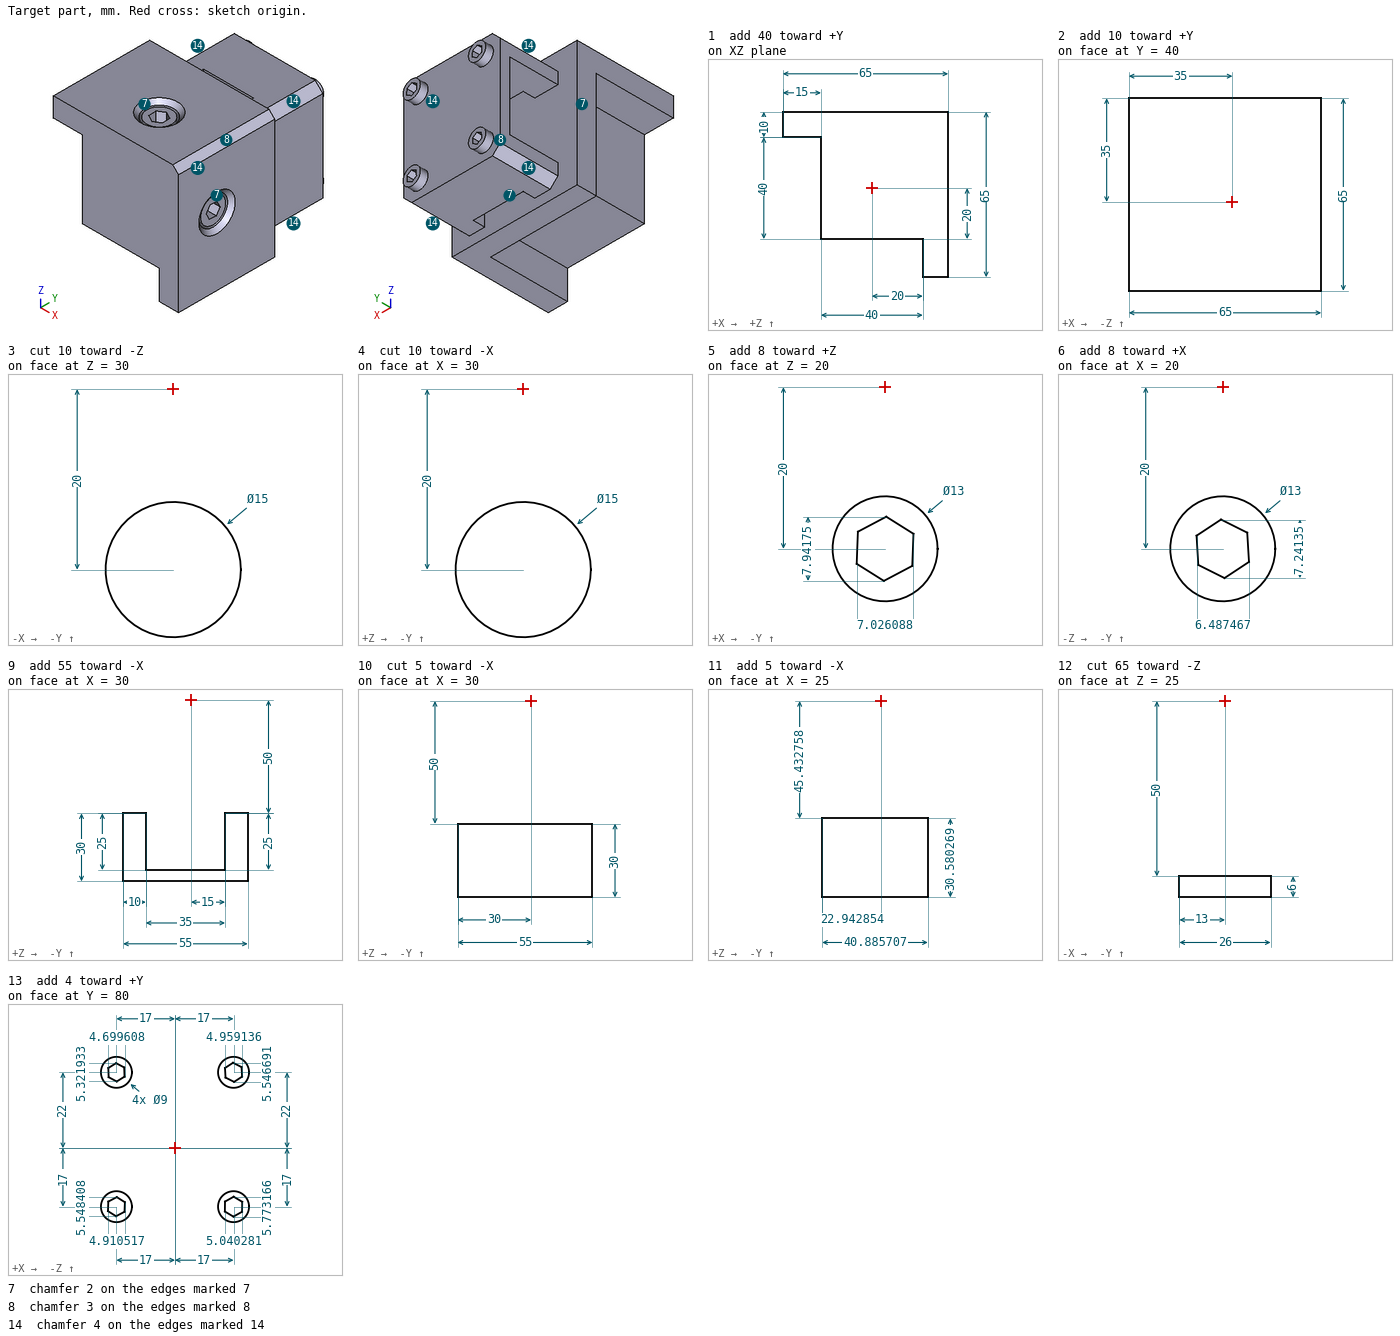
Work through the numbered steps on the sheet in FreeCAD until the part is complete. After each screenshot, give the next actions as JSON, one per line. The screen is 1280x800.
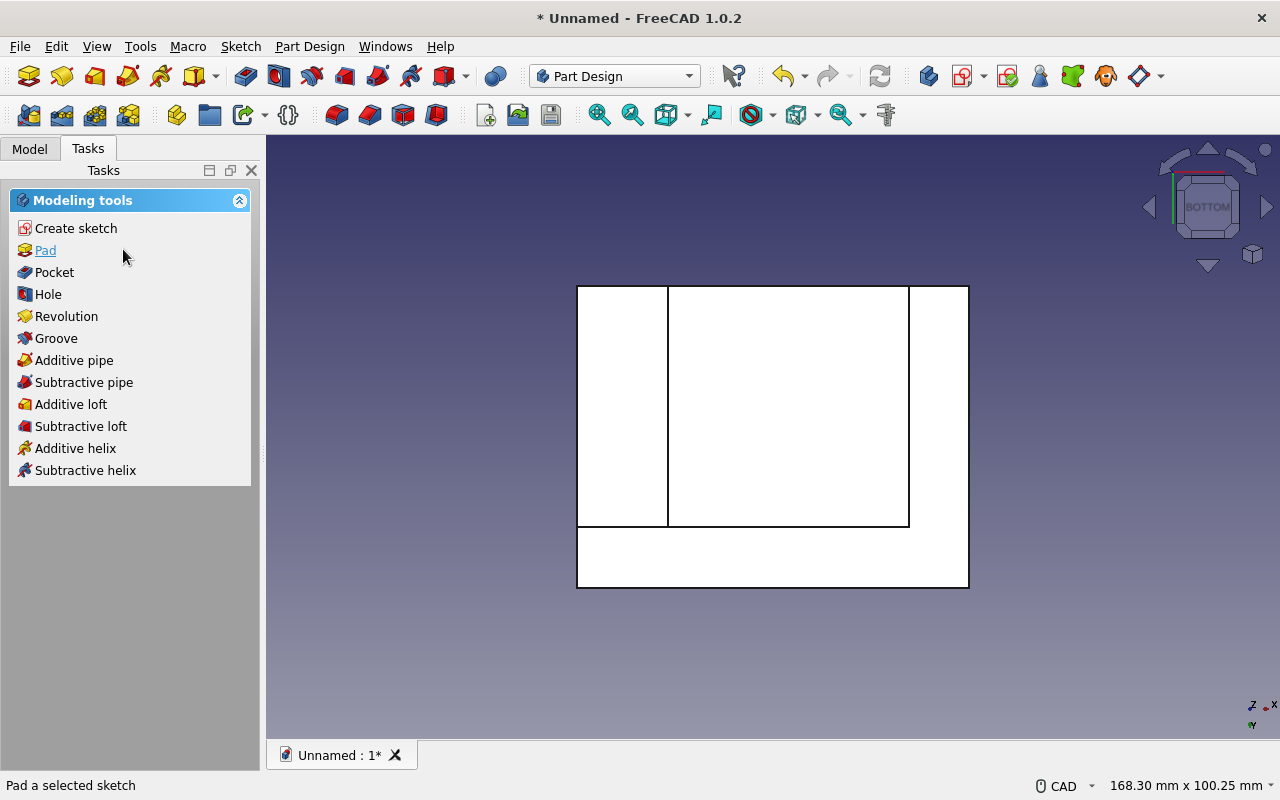
{"action": "left_click", "coordinate": [29, 76]}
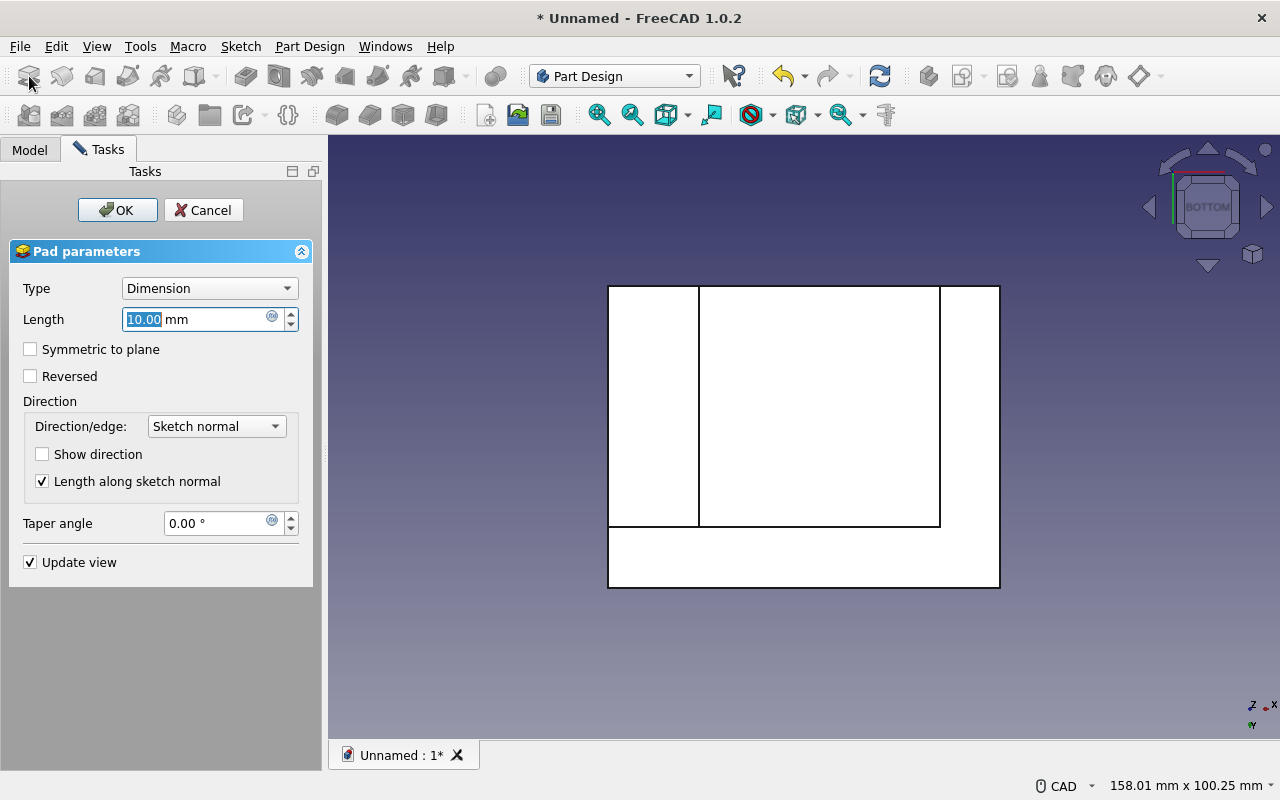
{"action": "type", "text": "8"}
{"action": "key", "text": "Tab"}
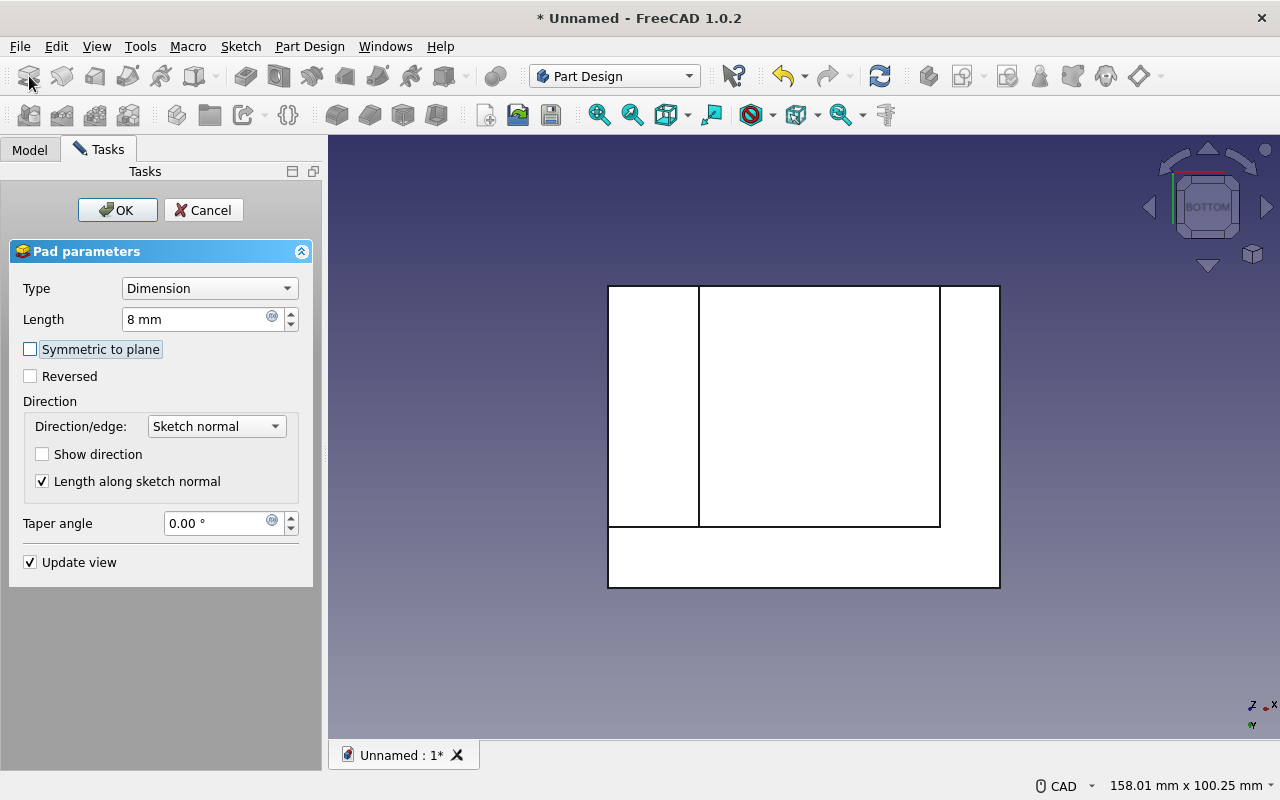
{"action": "left_click", "coordinate": [31, 376]}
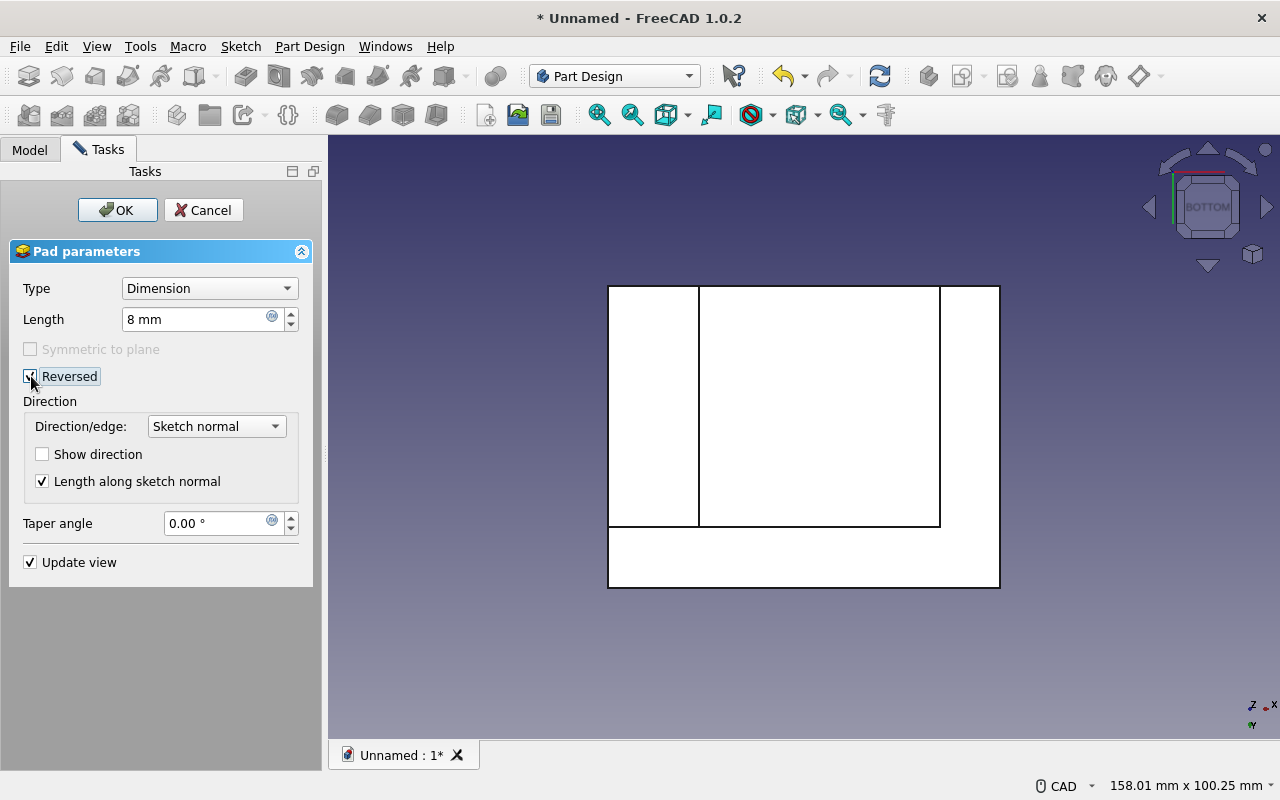
{"action": "left_click", "coordinate": [118, 210]}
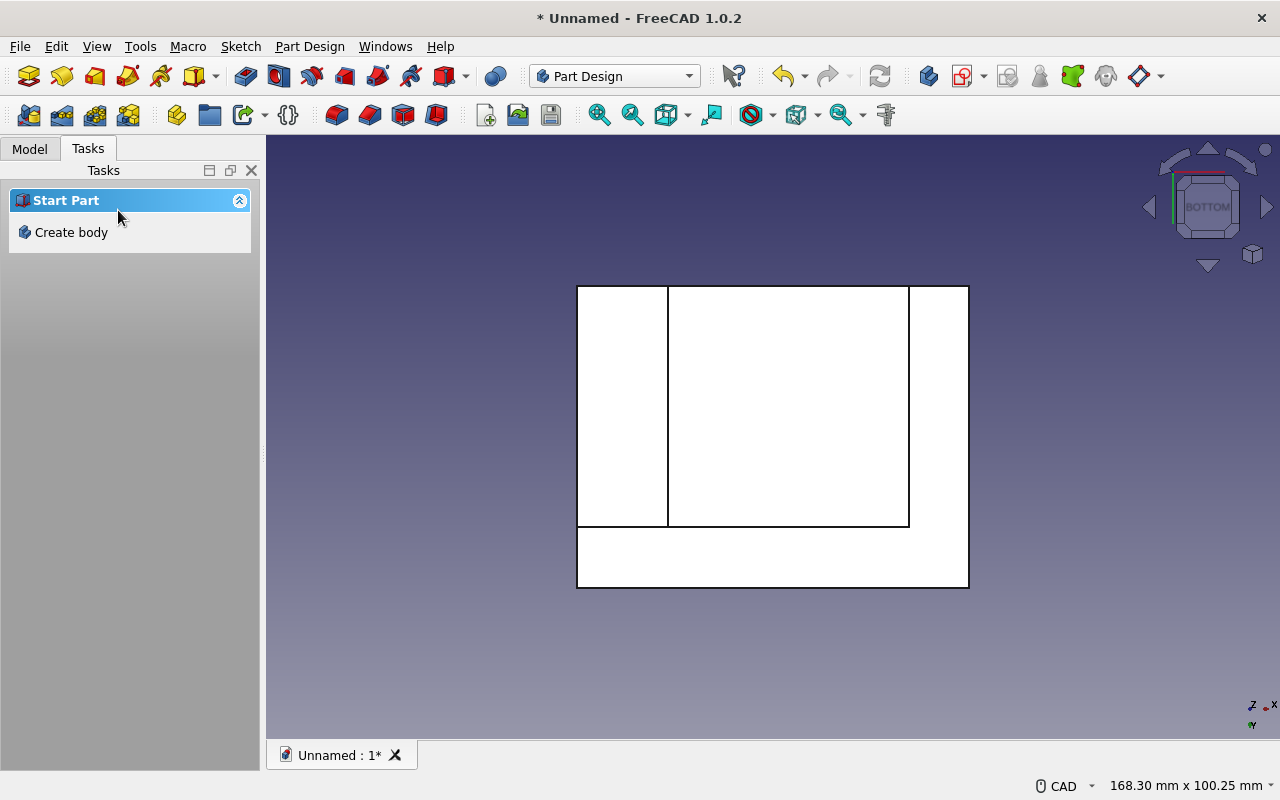
{"action": "key", "text": "6"}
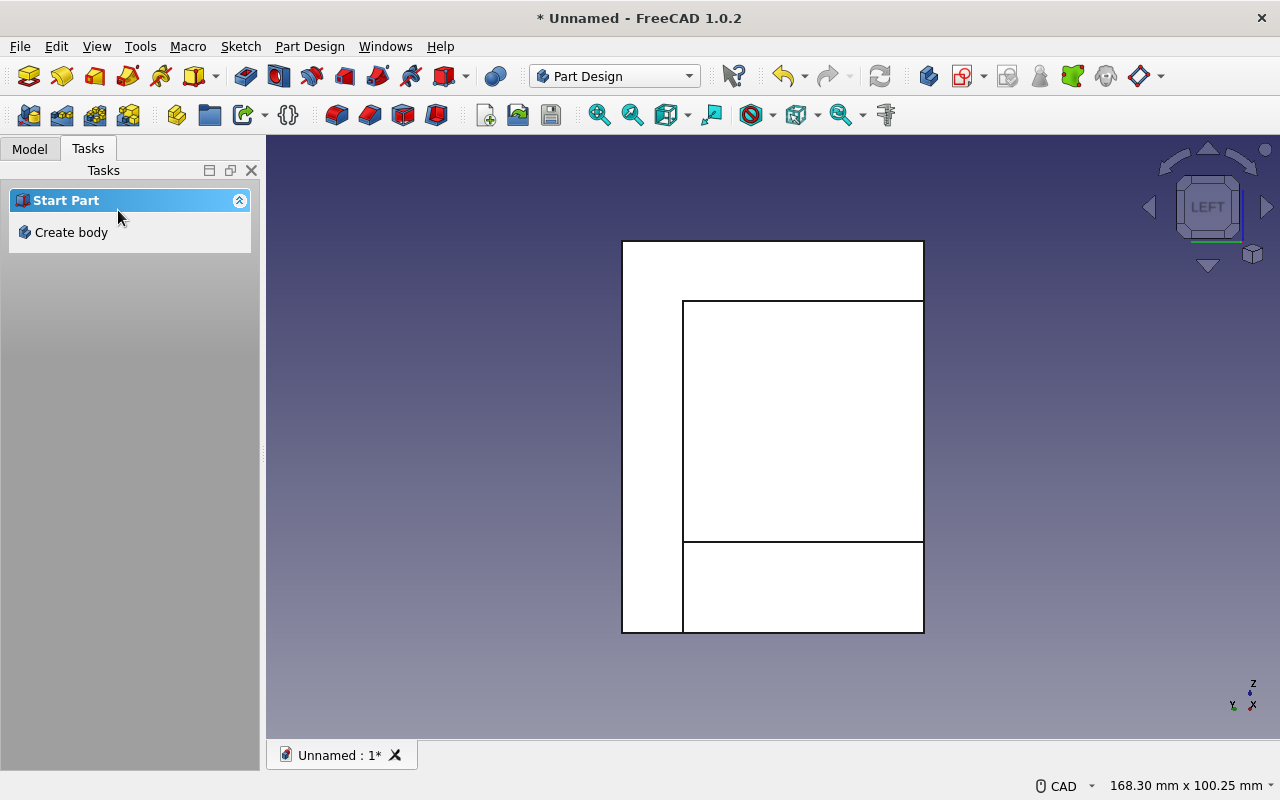
{"action": "left_click", "coordinate": [769, 587]}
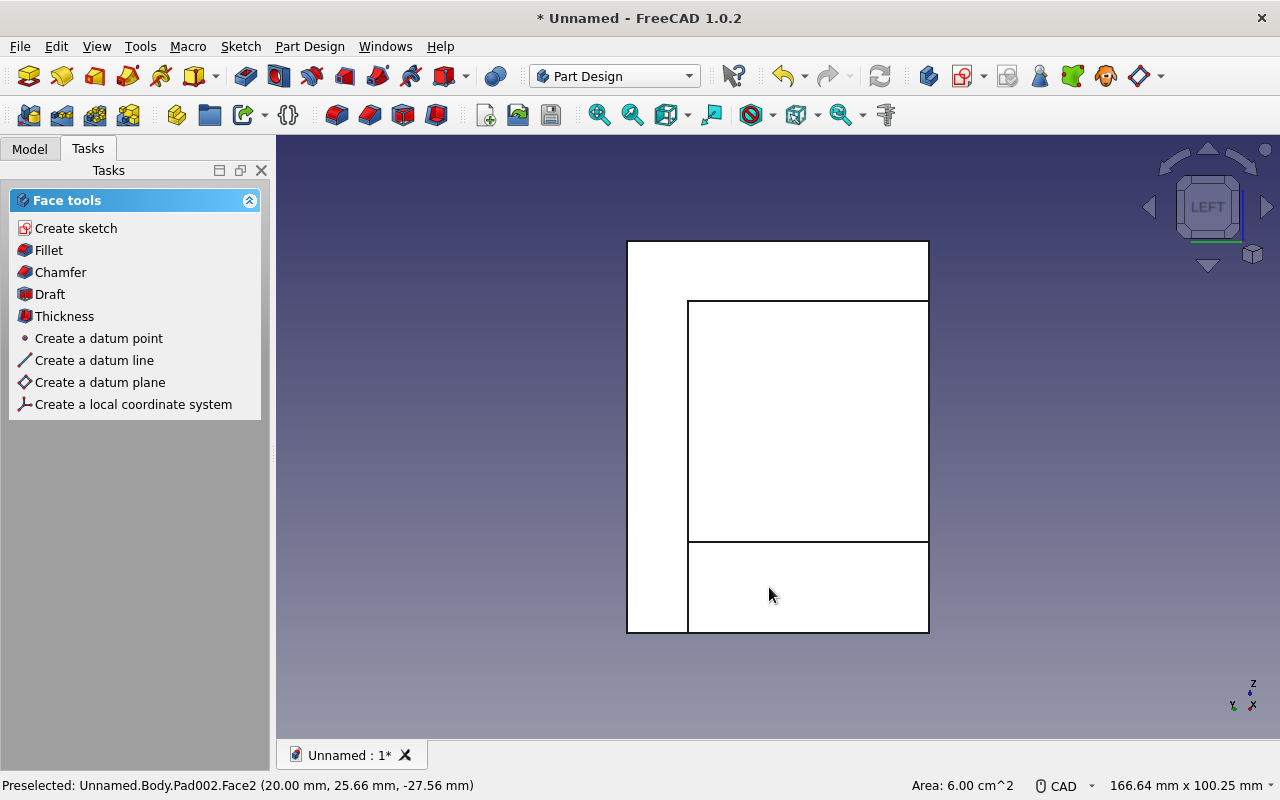
{"action": "left_click", "coordinate": [962, 76]}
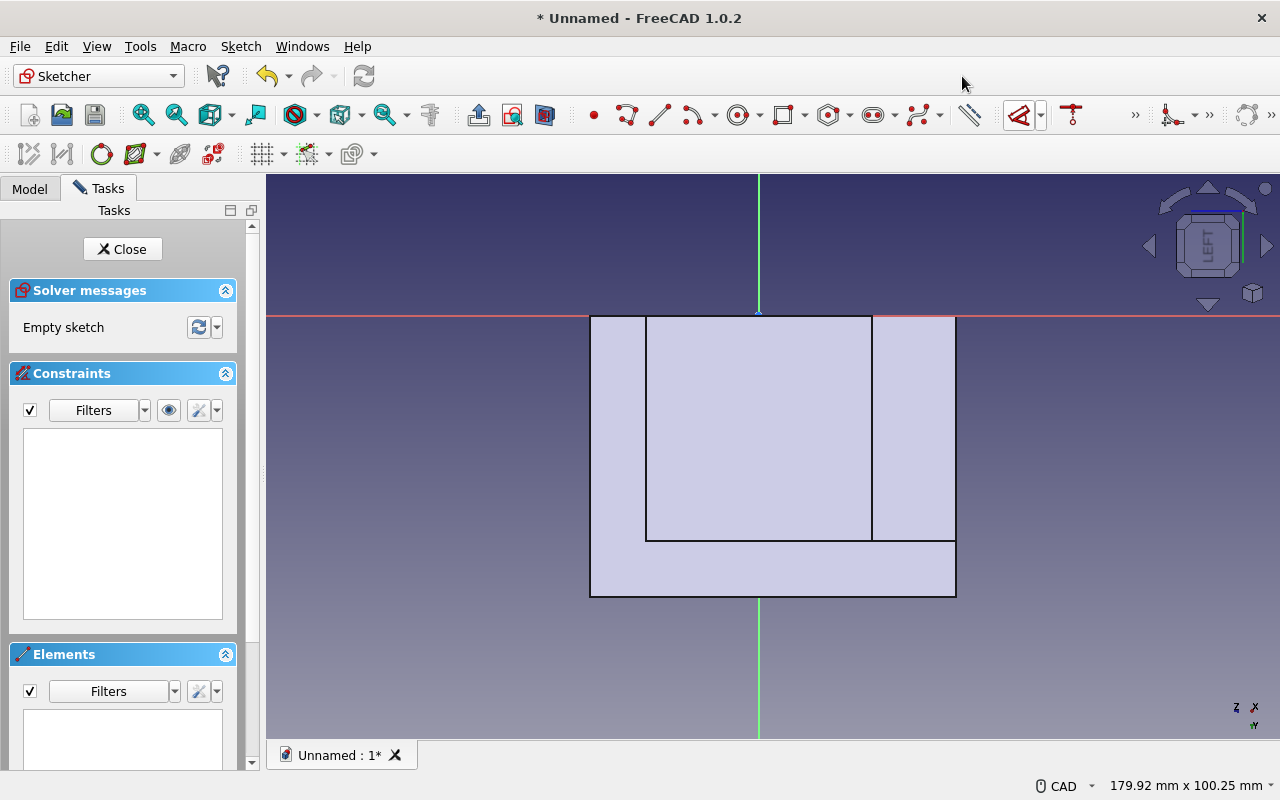
{"action": "scroll", "coordinate": [803, 336], "scroll_direction": "up", "scroll_amount": 4}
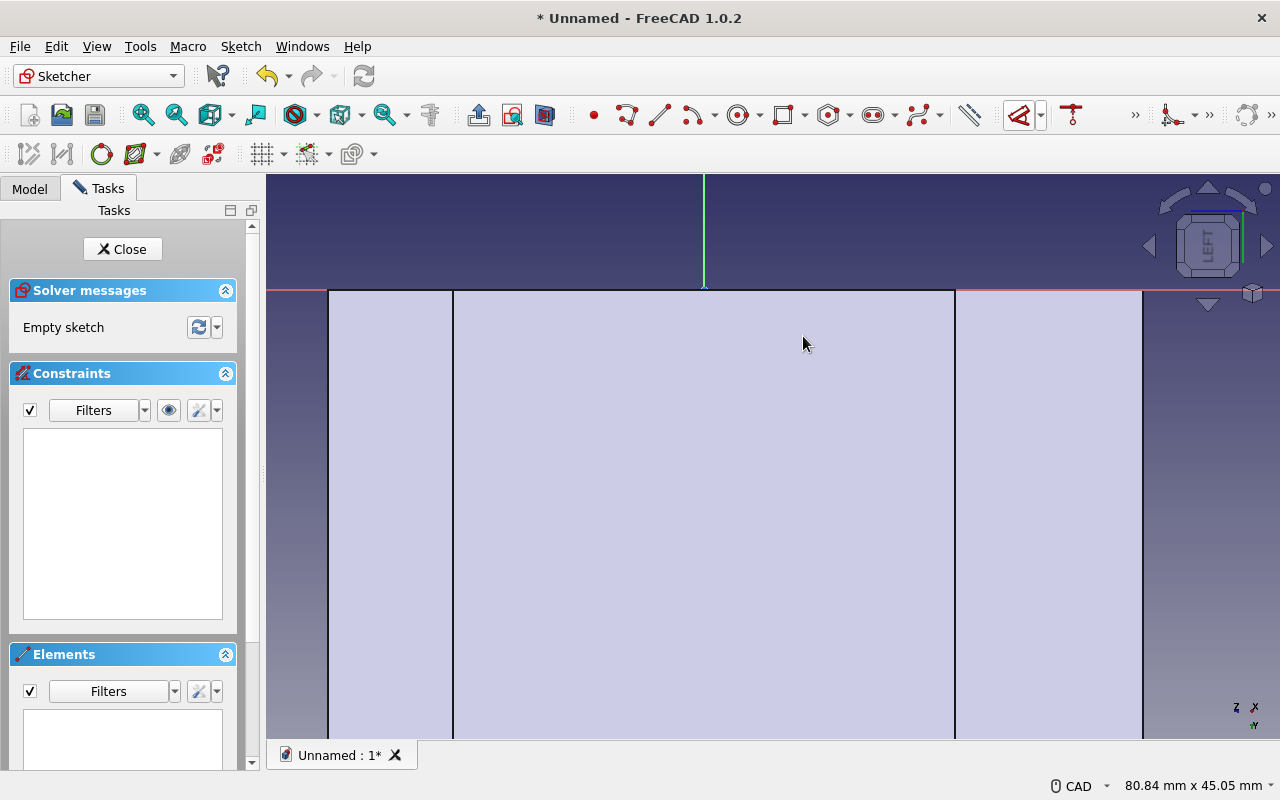
{"action": "left_click", "coordinate": [828, 116]}